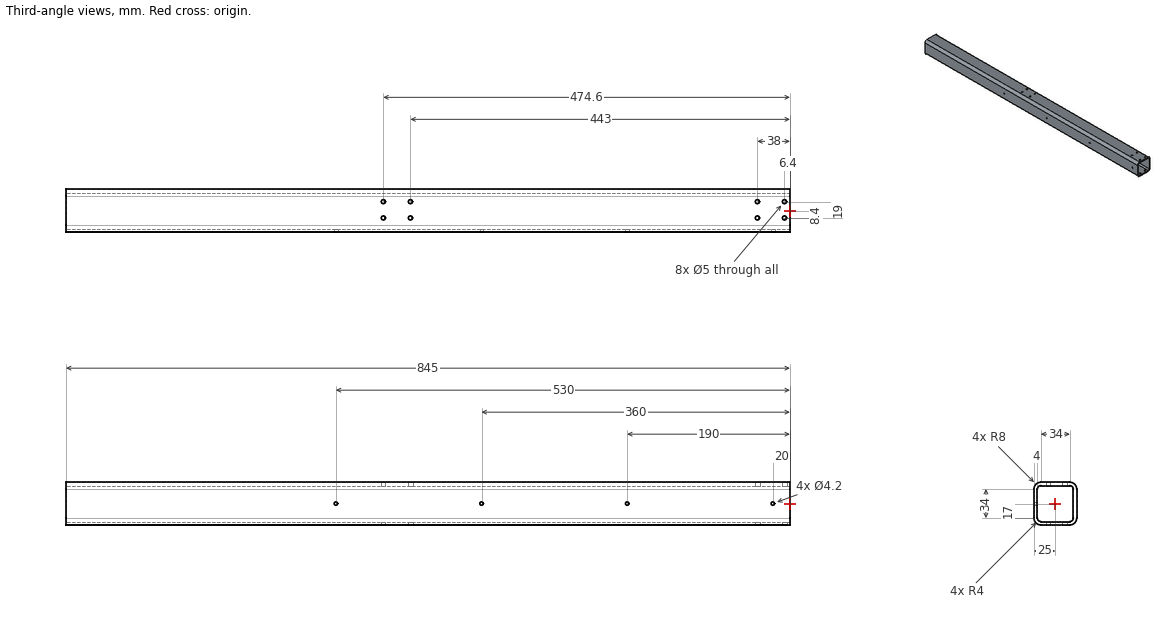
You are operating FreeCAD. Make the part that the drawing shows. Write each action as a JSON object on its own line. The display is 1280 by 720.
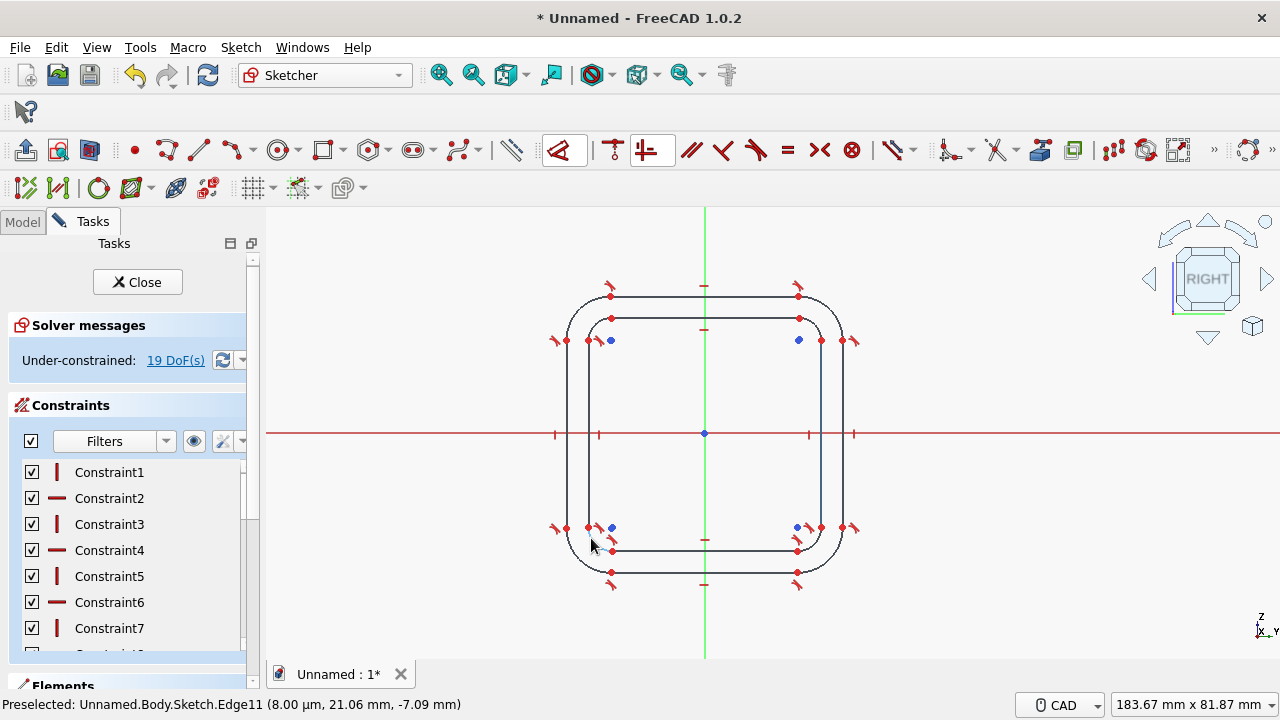
{"action": "scroll", "coordinate": [819, 331], "scroll_direction": "up", "scroll_amount": 2}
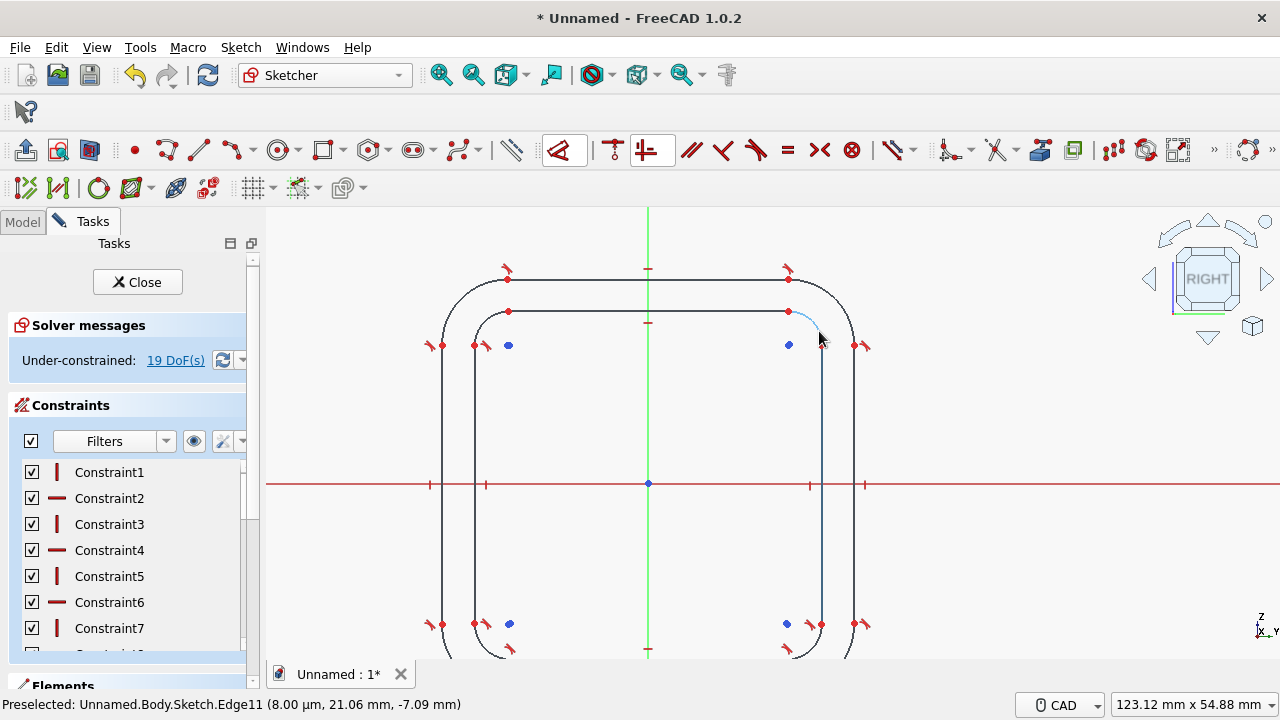
{"action": "left_click", "coordinate": [819, 330]}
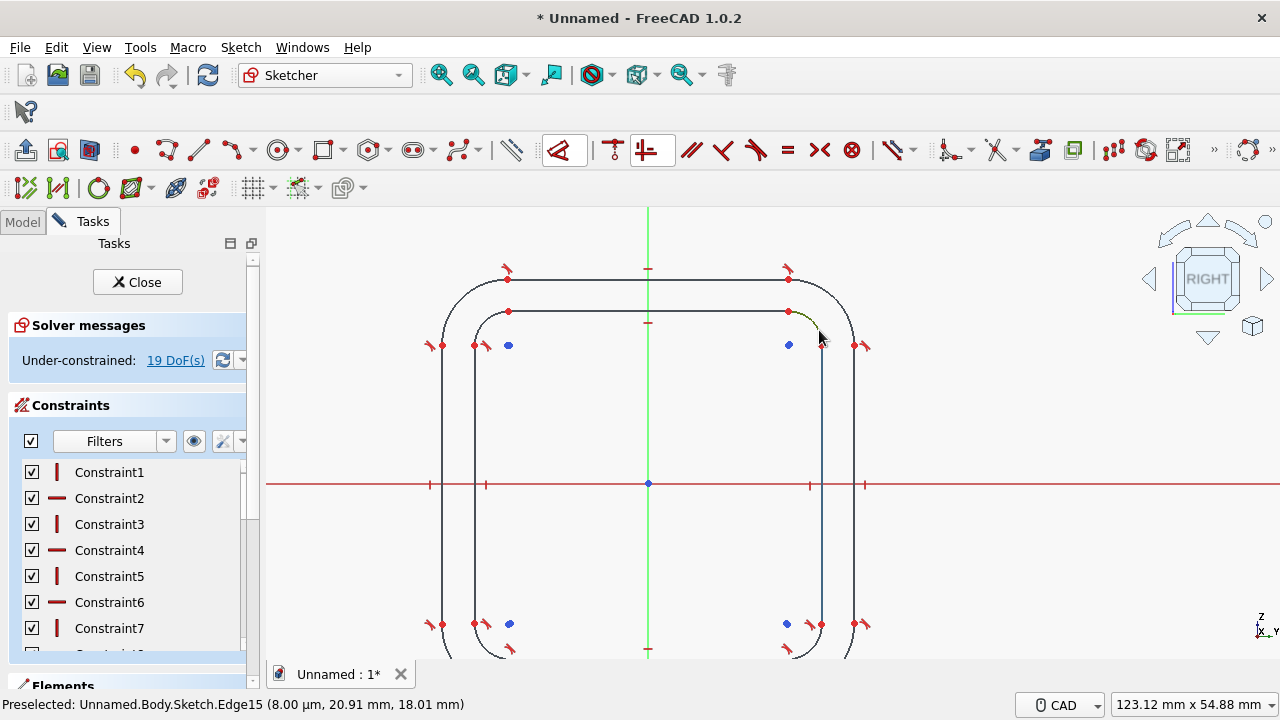
{"action": "left_click", "coordinate": [756, 150]}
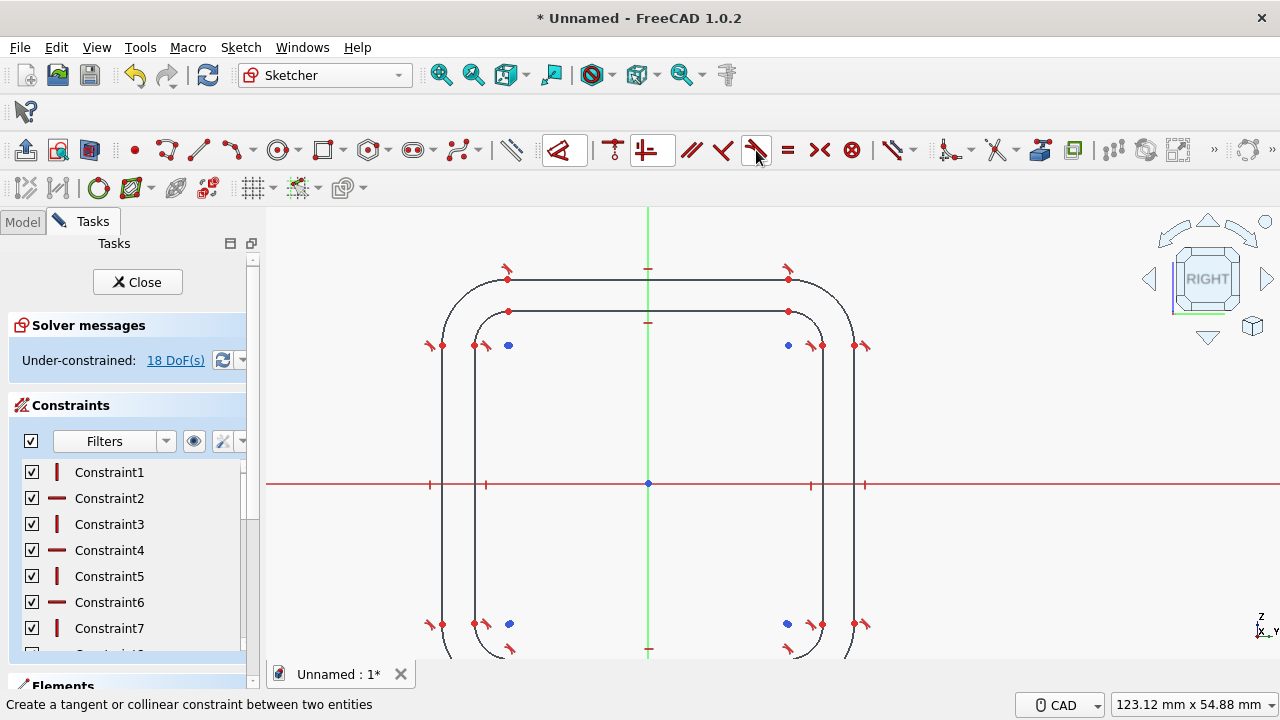
{"action": "left_click", "coordinate": [705, 311]}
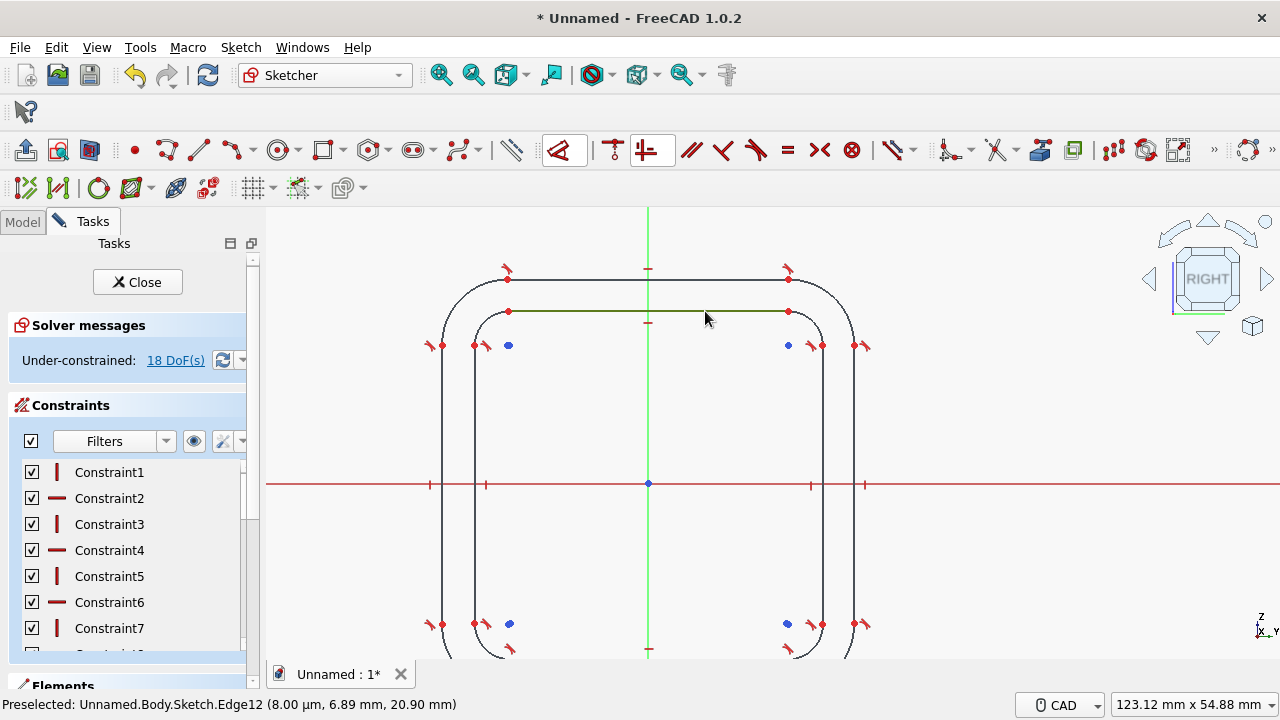
{"action": "left_click", "coordinate": [819, 330]}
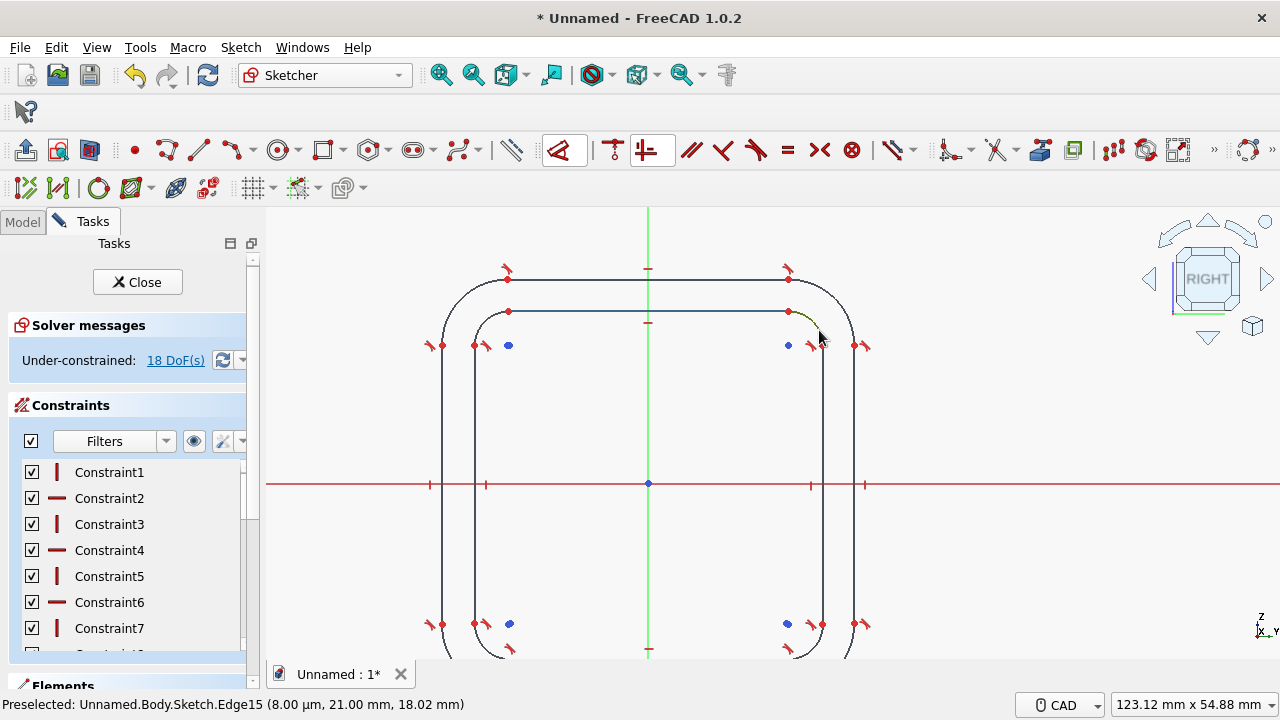
{"action": "left_click", "coordinate": [756, 150]}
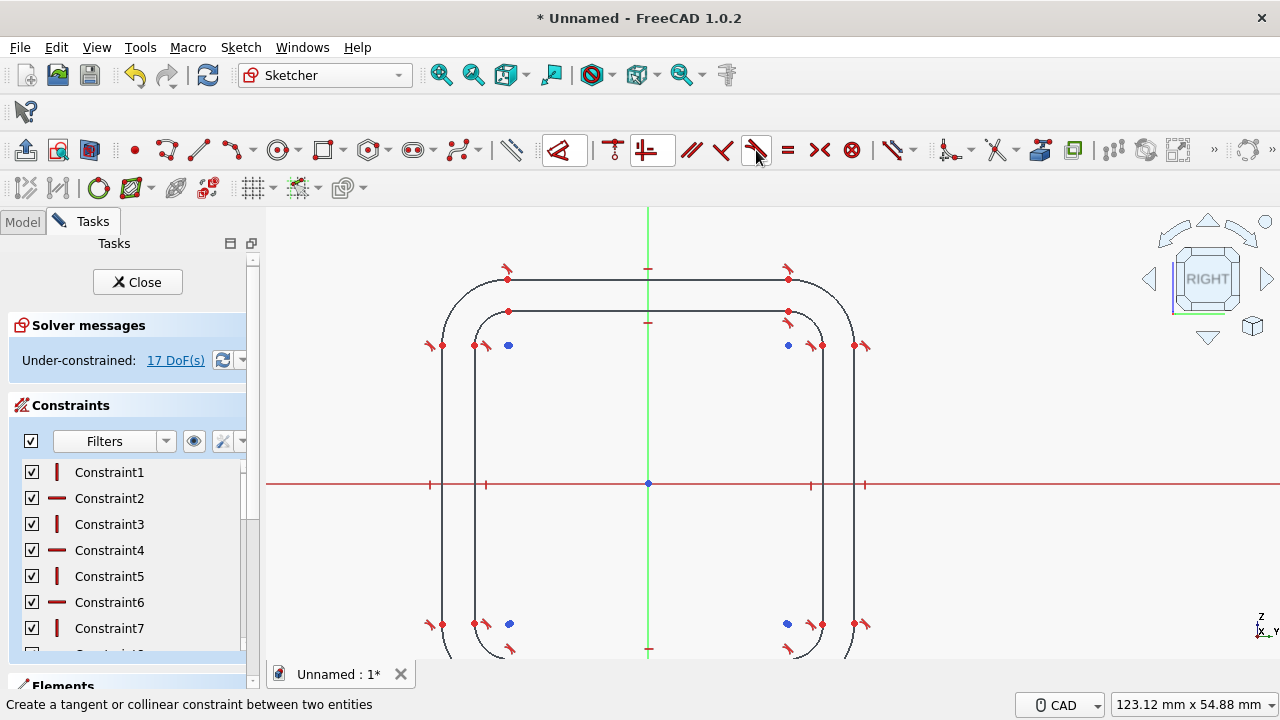
{"action": "left_click", "coordinate": [705, 311]}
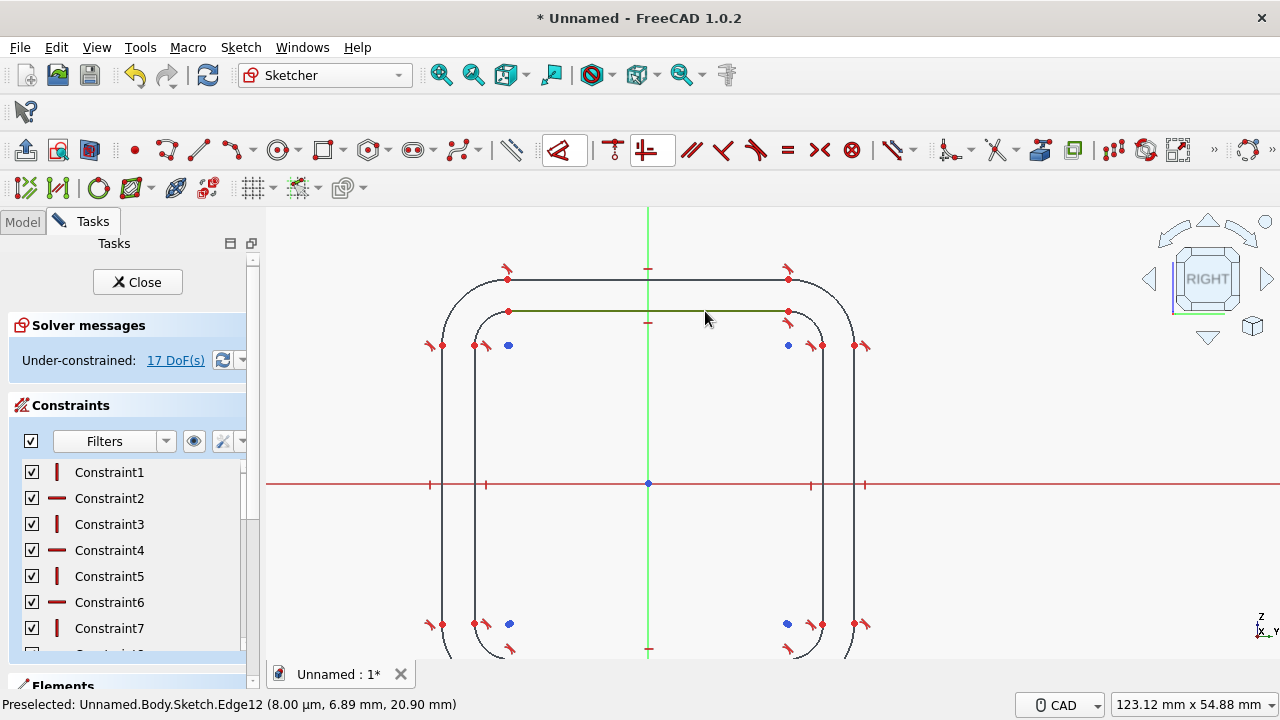
{"action": "left_click", "coordinate": [493, 315]}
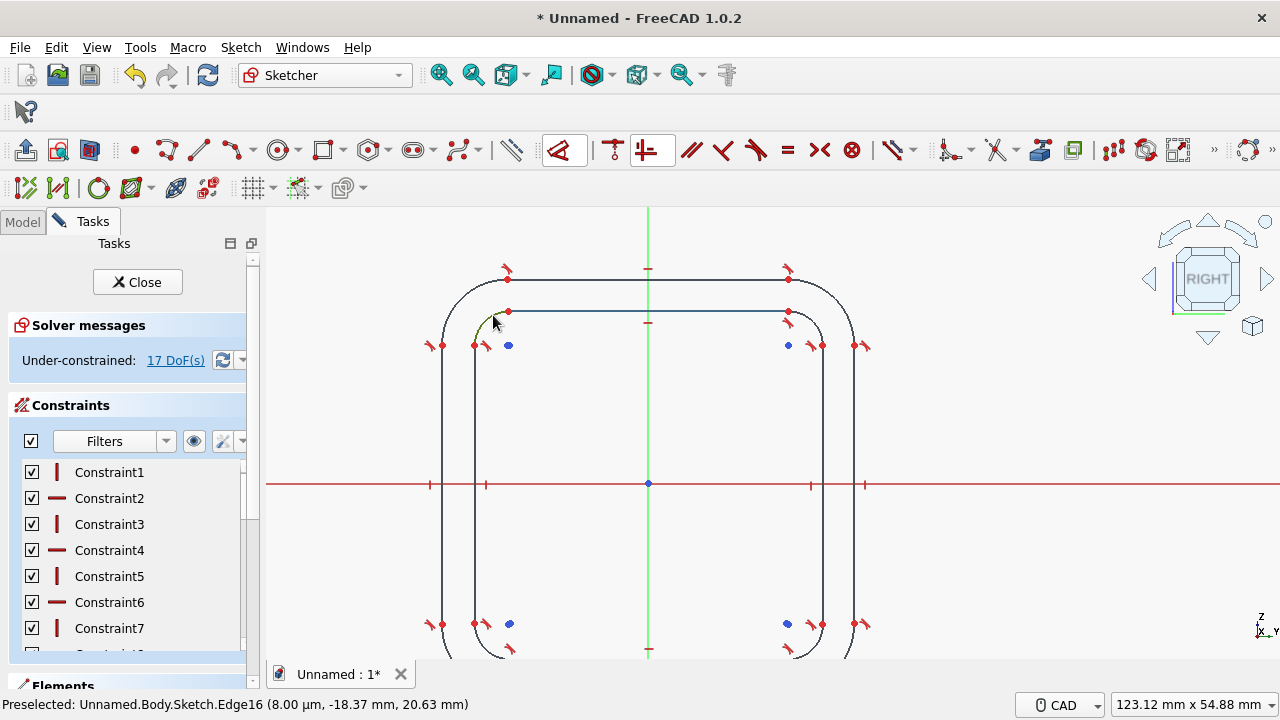
{"action": "left_click", "coordinate": [756, 150]}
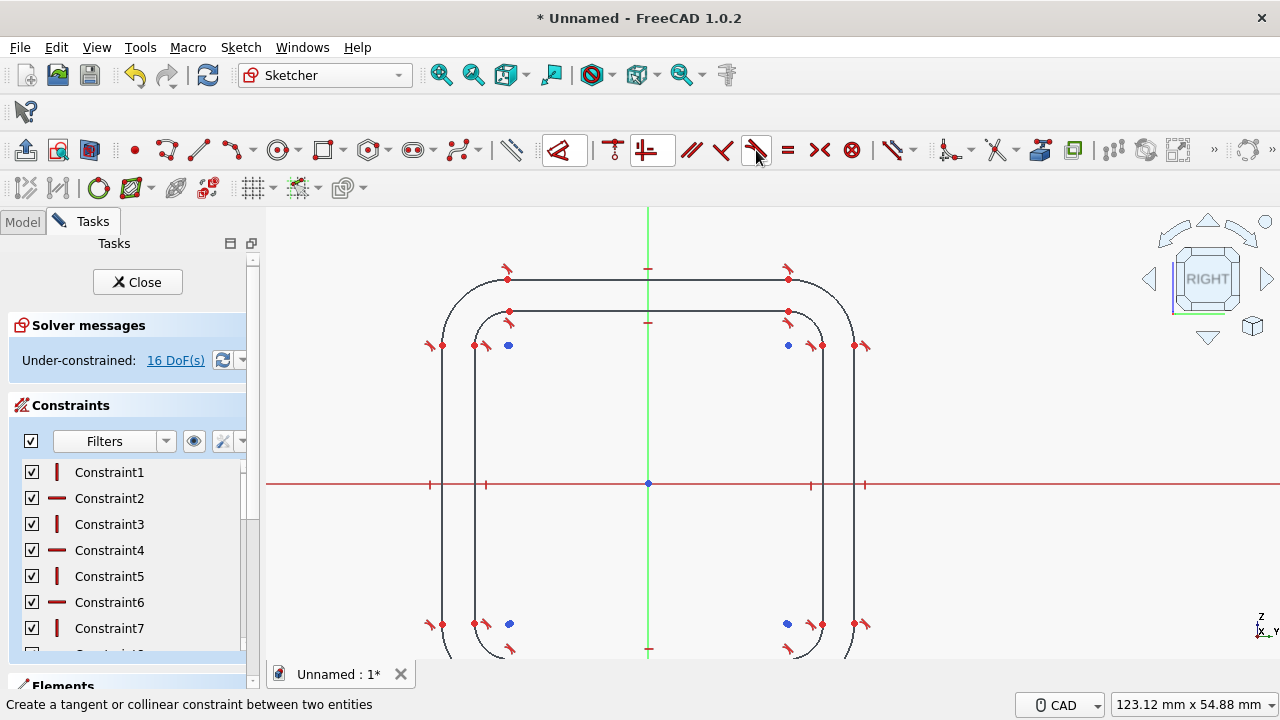
{"action": "scroll", "coordinate": [819, 330], "scroll_direction": "down", "scroll_amount": 2}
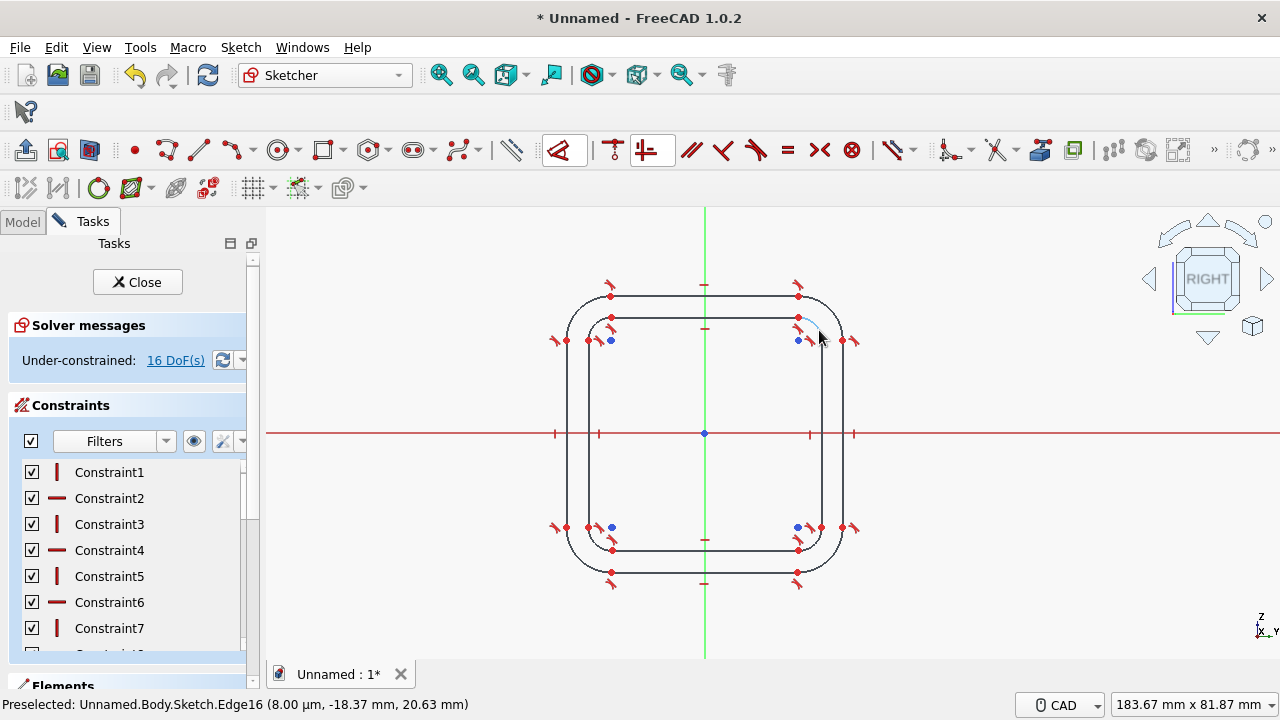
{"action": "left_click", "coordinate": [571, 548]}